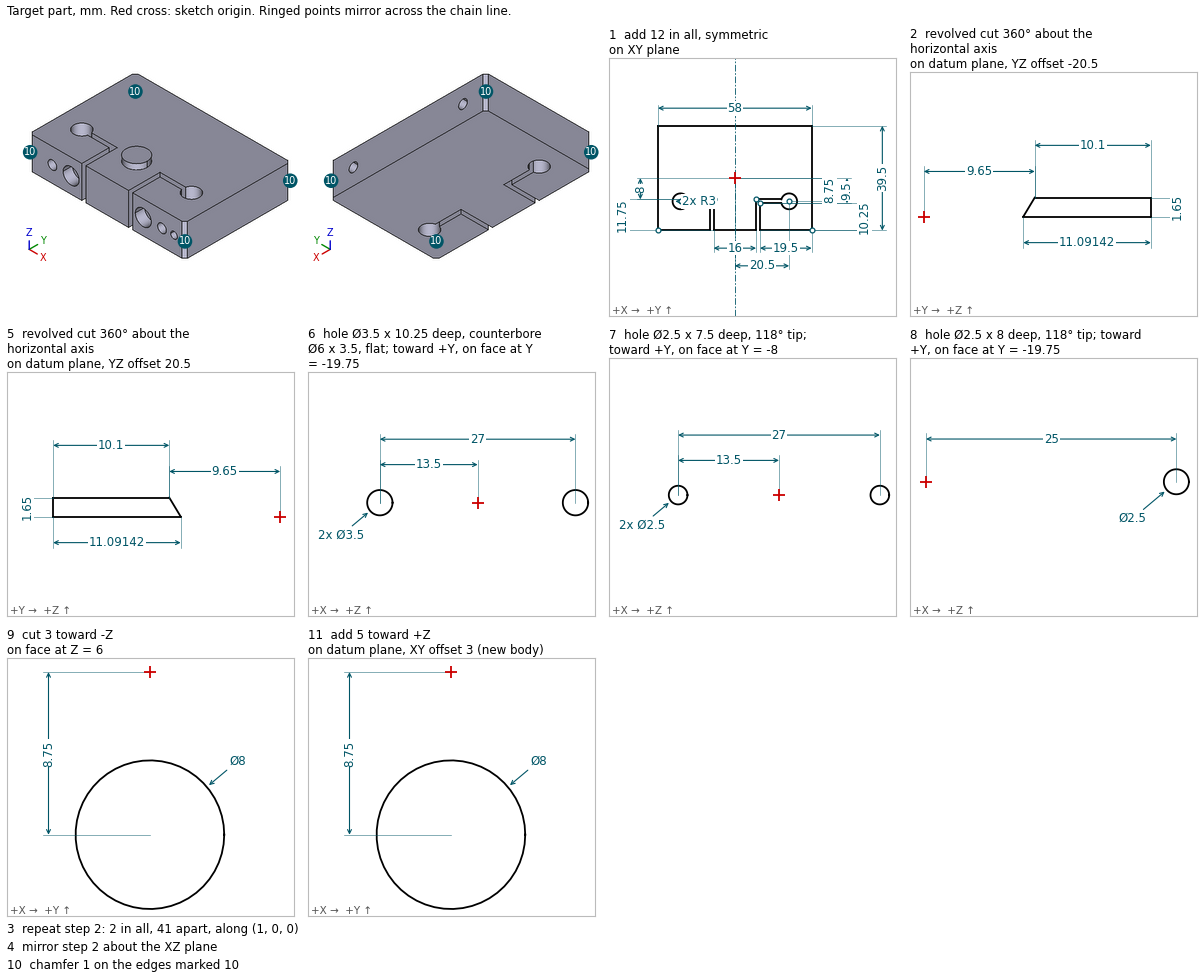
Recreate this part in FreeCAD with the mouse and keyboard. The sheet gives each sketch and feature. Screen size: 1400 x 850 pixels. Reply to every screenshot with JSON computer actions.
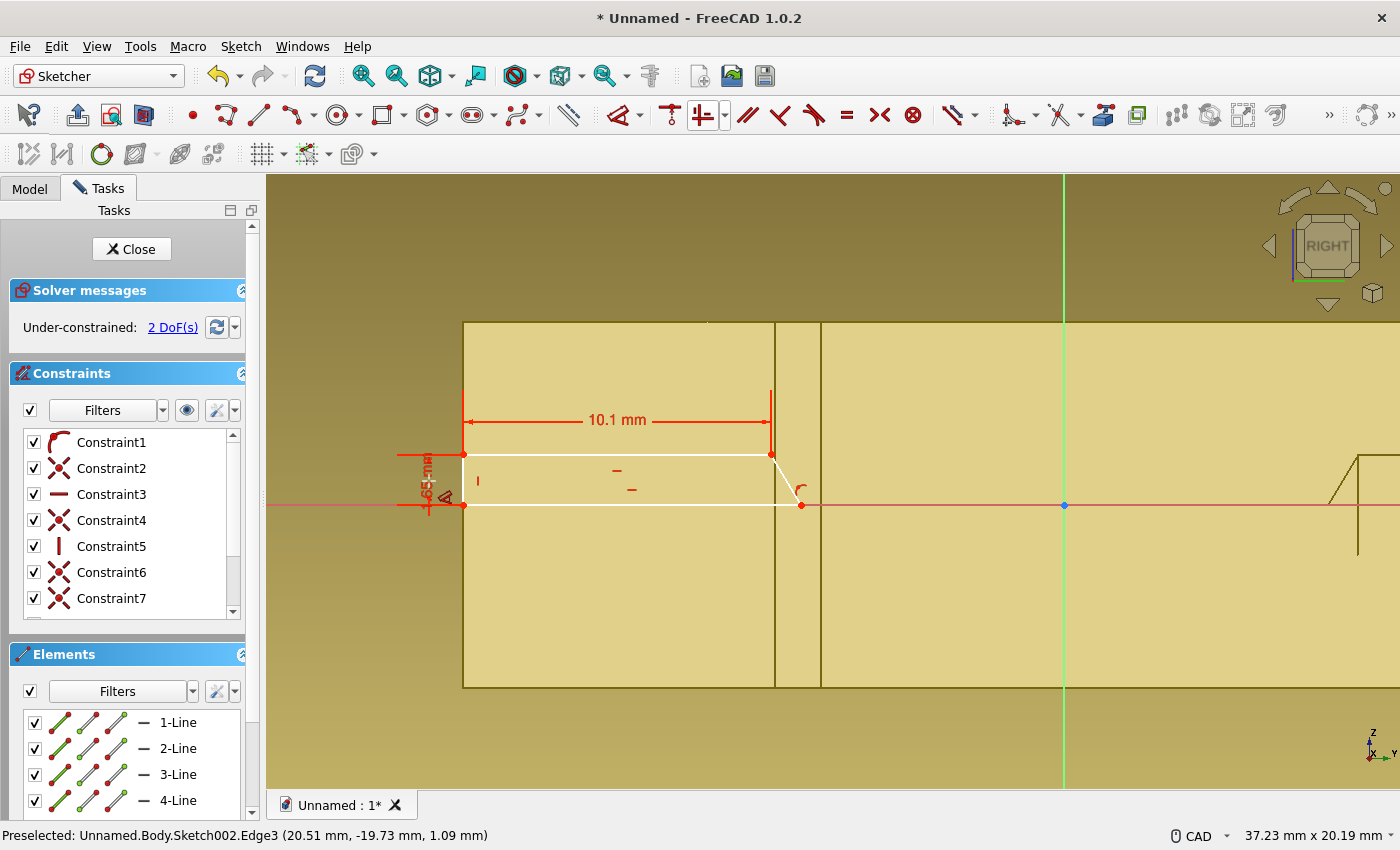
{"action": "left_click", "coordinate": [771, 455]}
{"action": "left_click", "coordinate": [918, 539]}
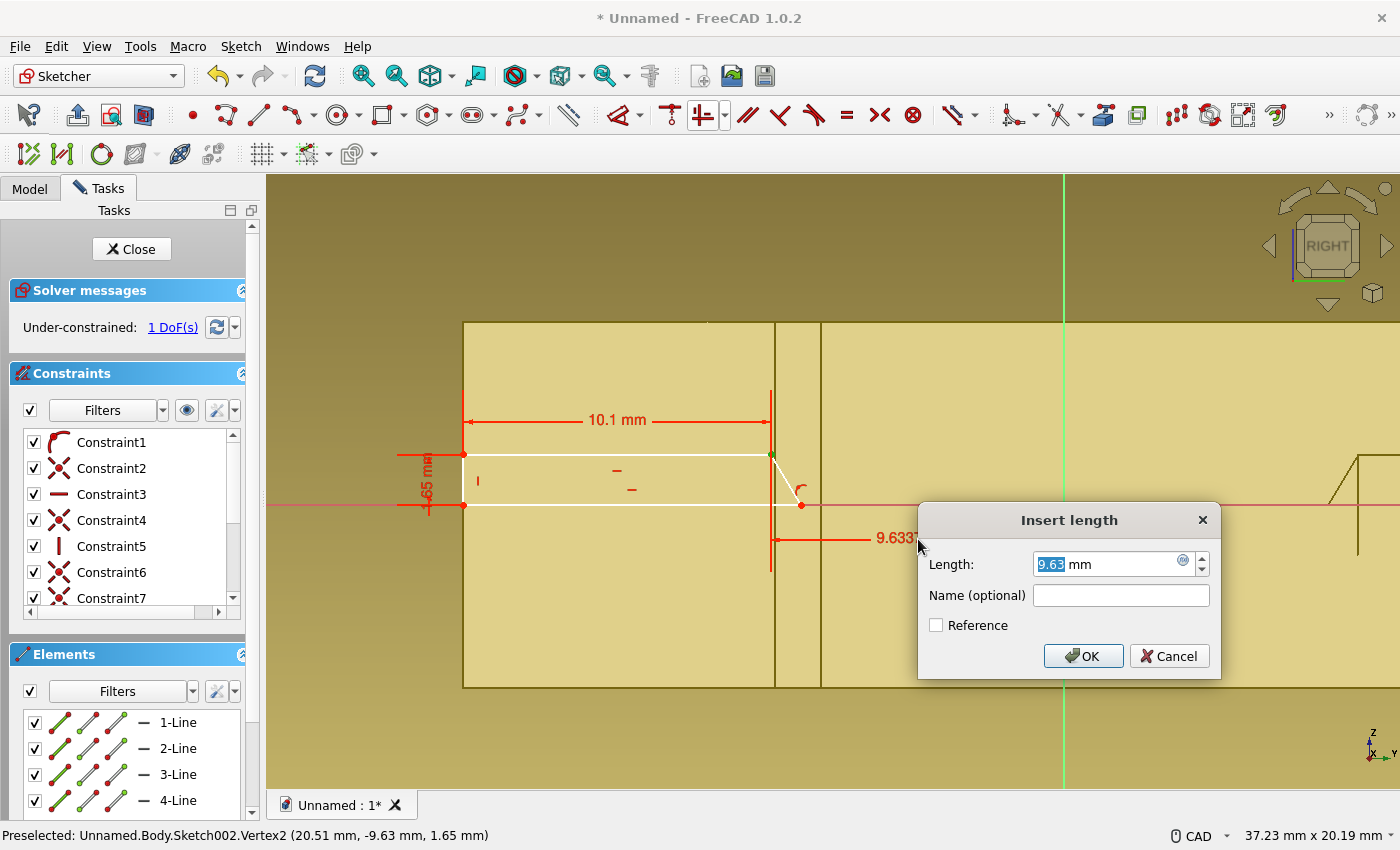
{"action": "type", "text": "9.65"}
{"action": "key", "text": "Return"}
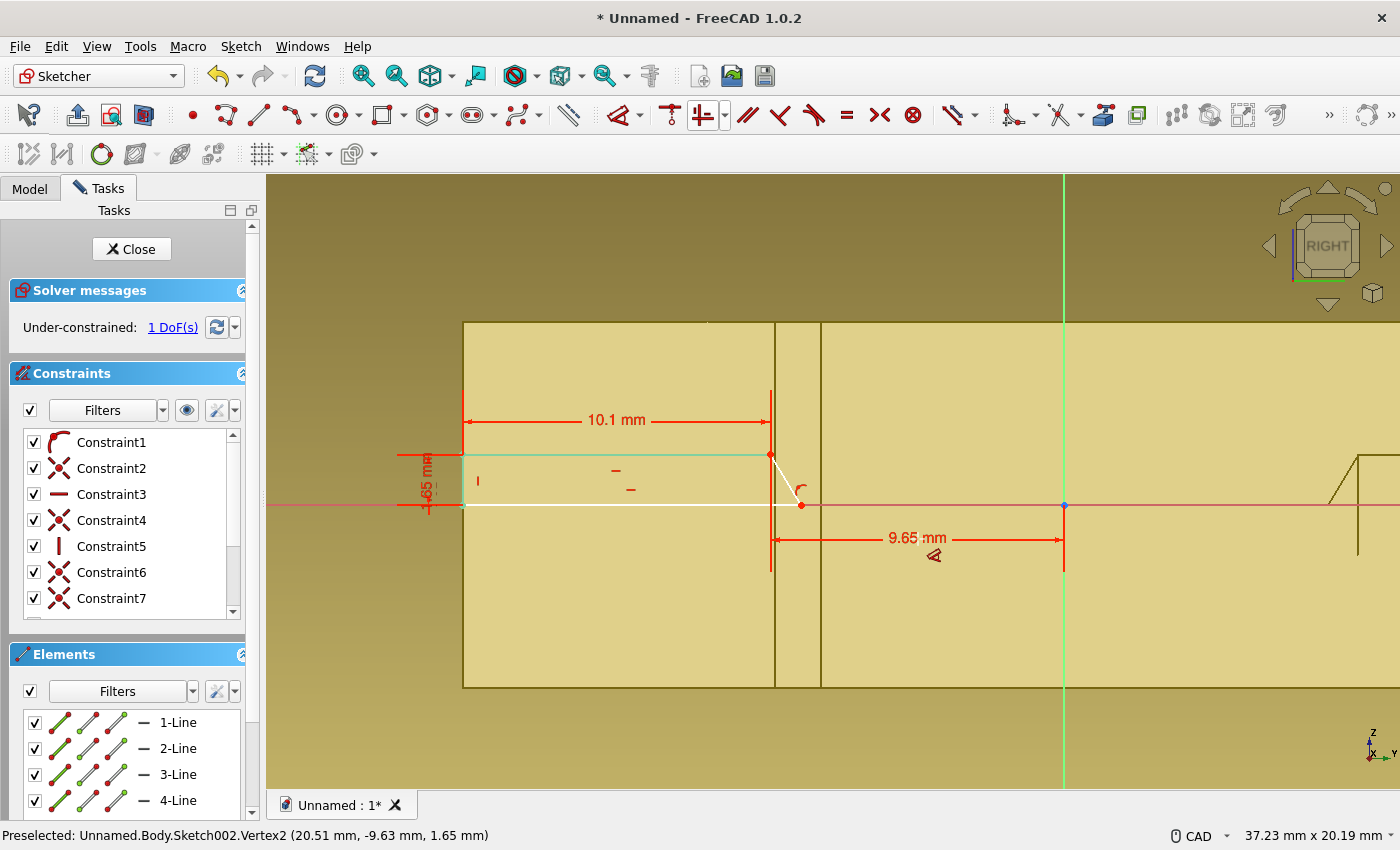
{"action": "left_click", "coordinate": [564, 505]}
{"action": "left_click", "coordinate": [632, 539]}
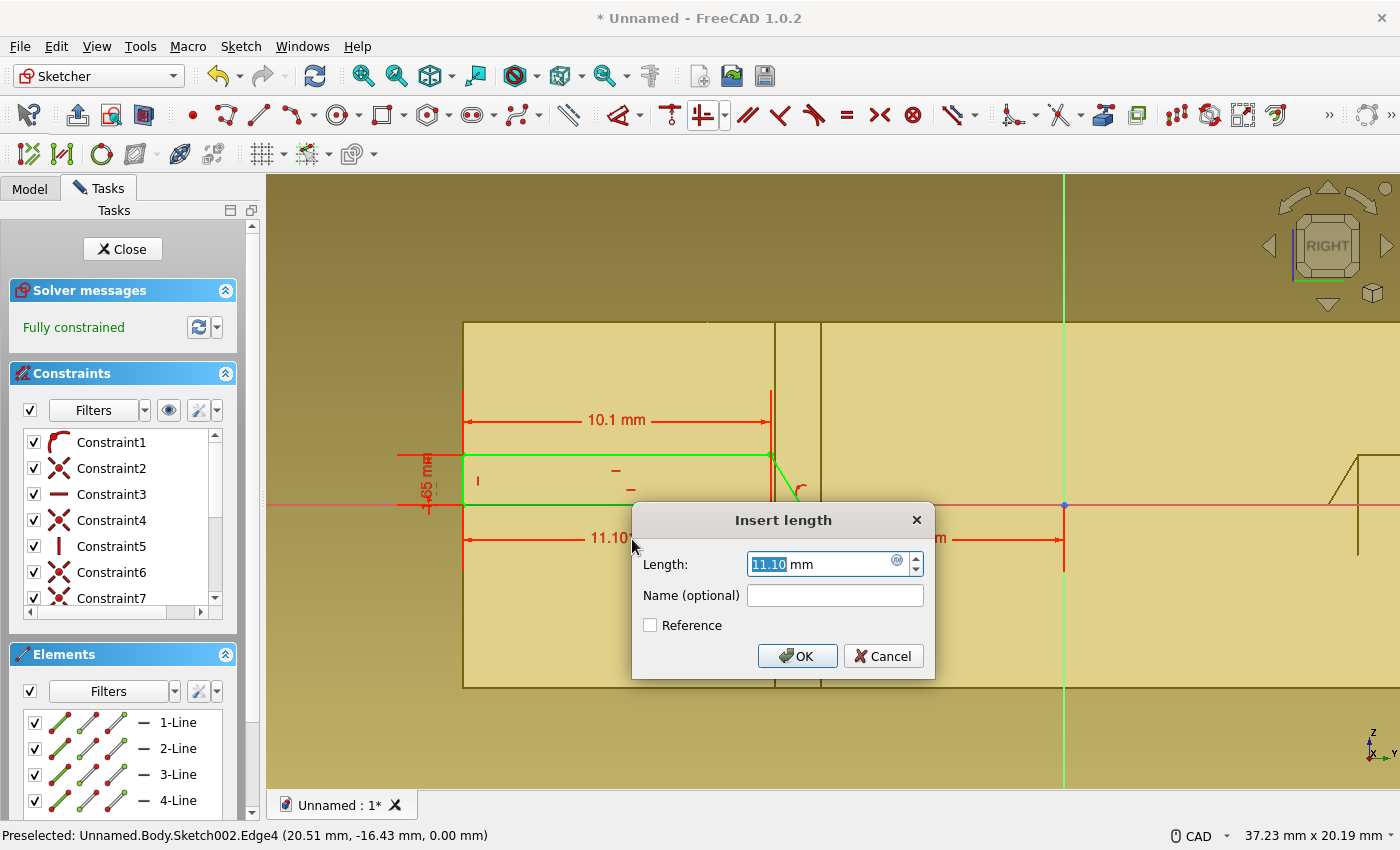
{"action": "type", "text": "11.09142"}
{"action": "key", "text": "Return"}
{"action": "key", "text": "Escape"}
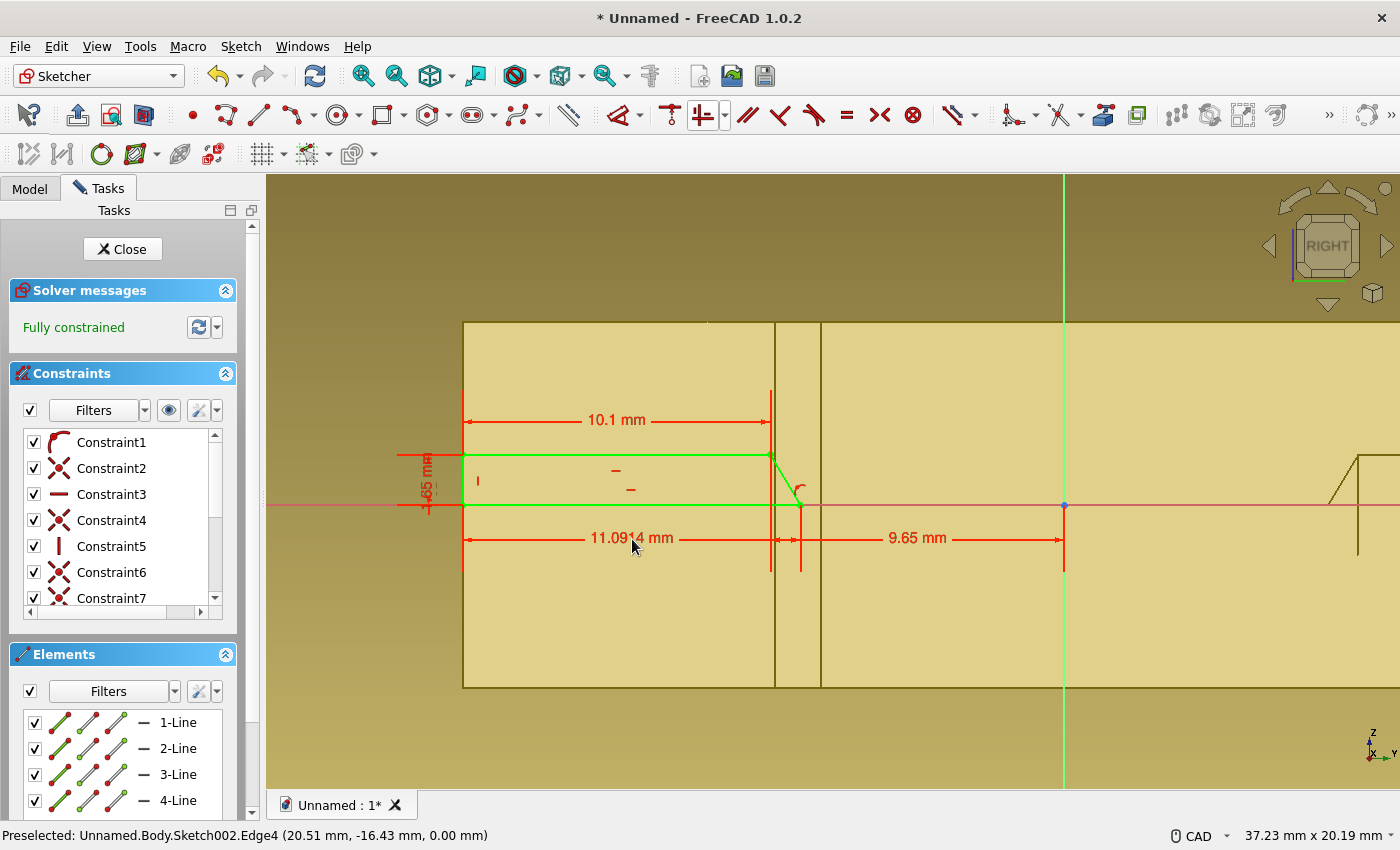
{"action": "left_click", "coordinate": [123, 249]}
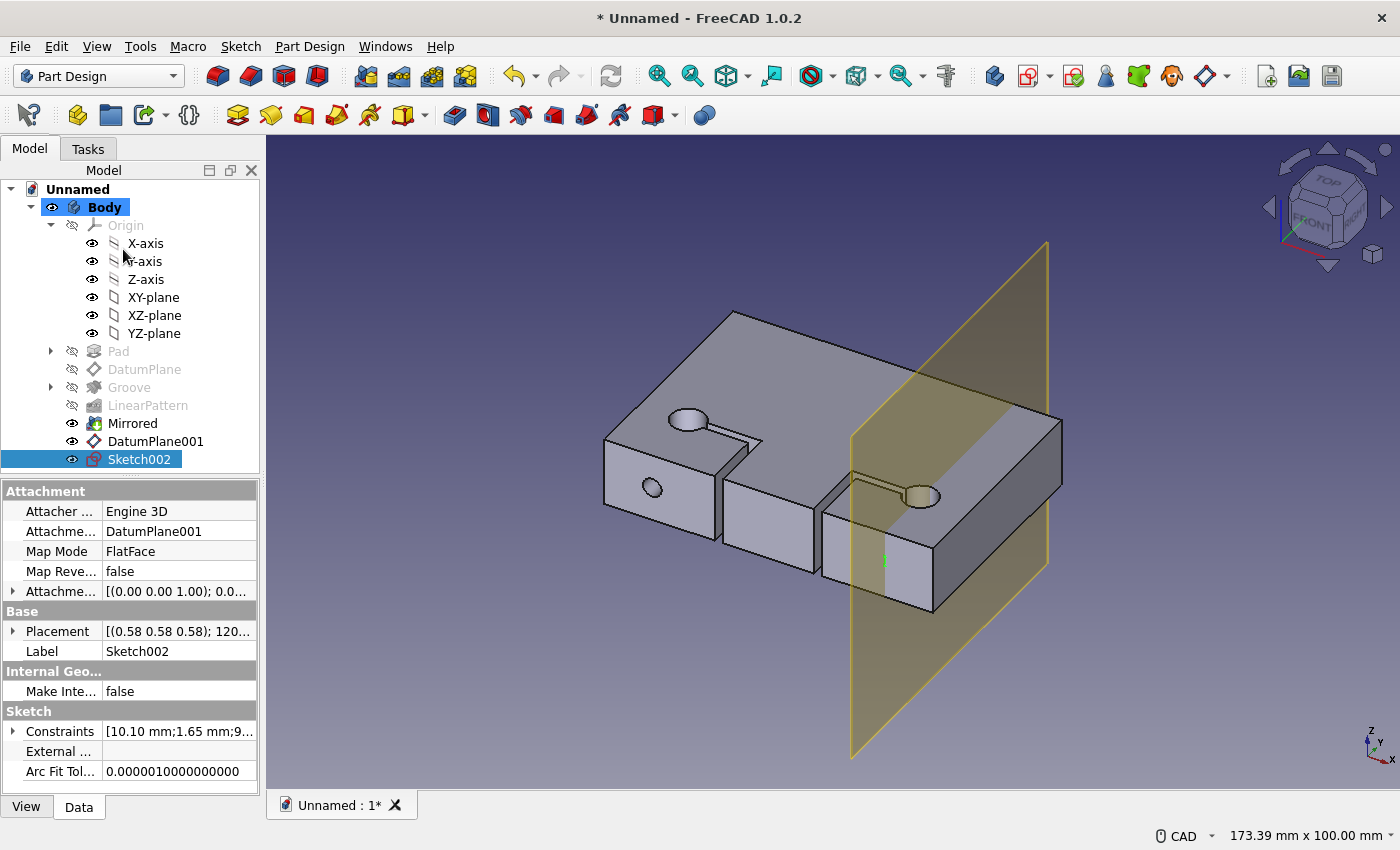
{"action": "left_click", "coordinate": [521, 116]}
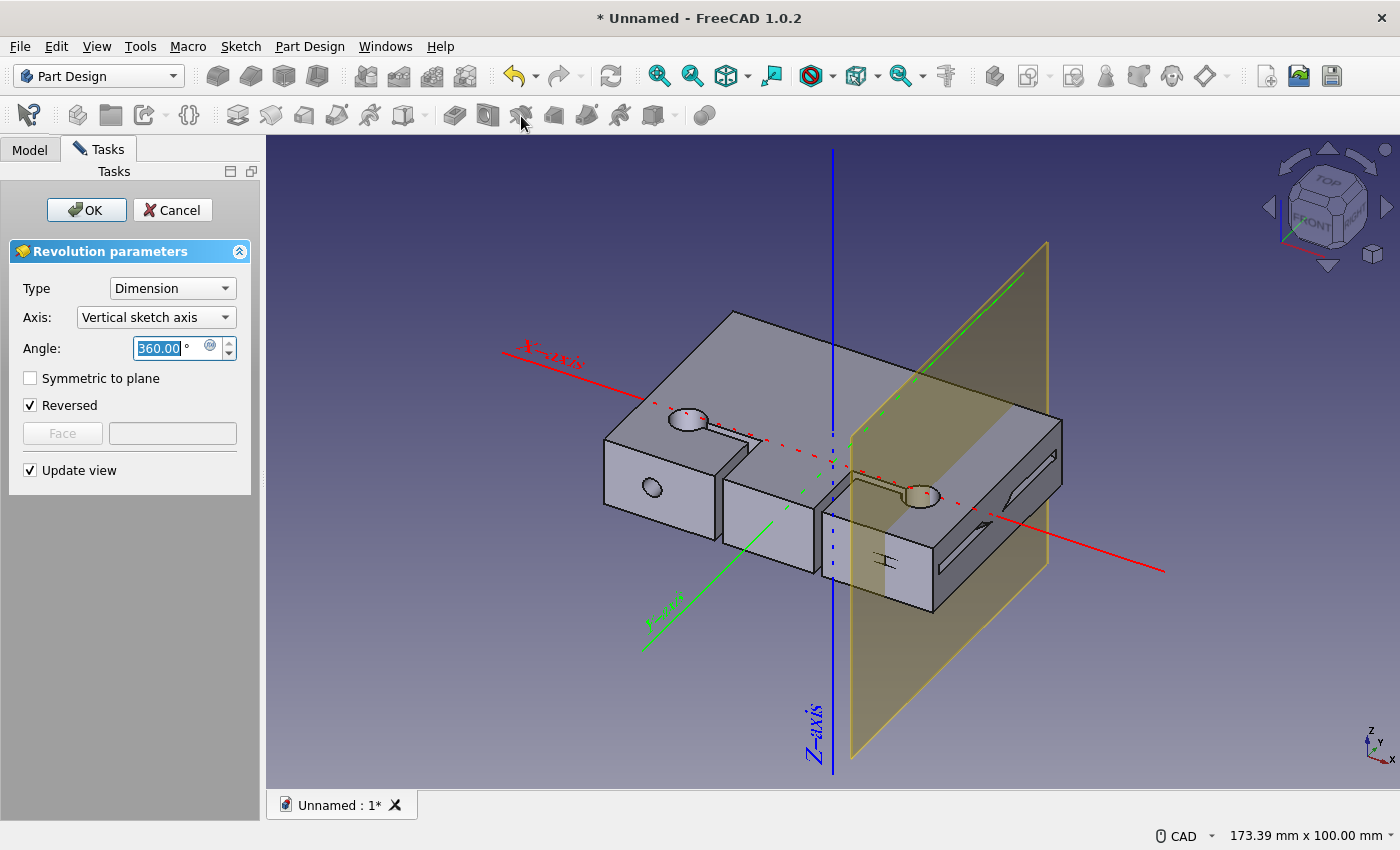
{"action": "left_click", "coordinate": [157, 318]}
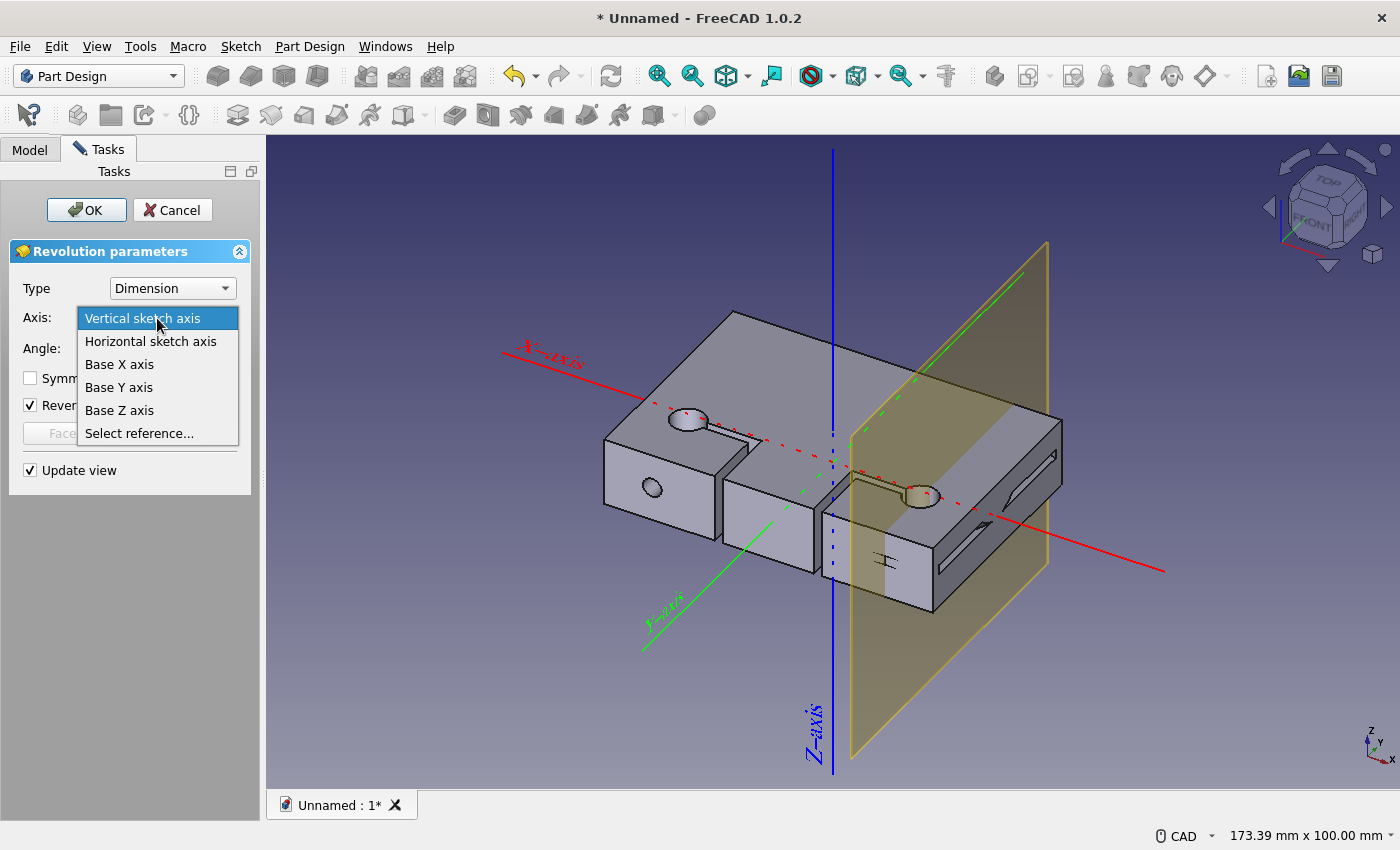
{"action": "left_click", "coordinate": [156, 342]}